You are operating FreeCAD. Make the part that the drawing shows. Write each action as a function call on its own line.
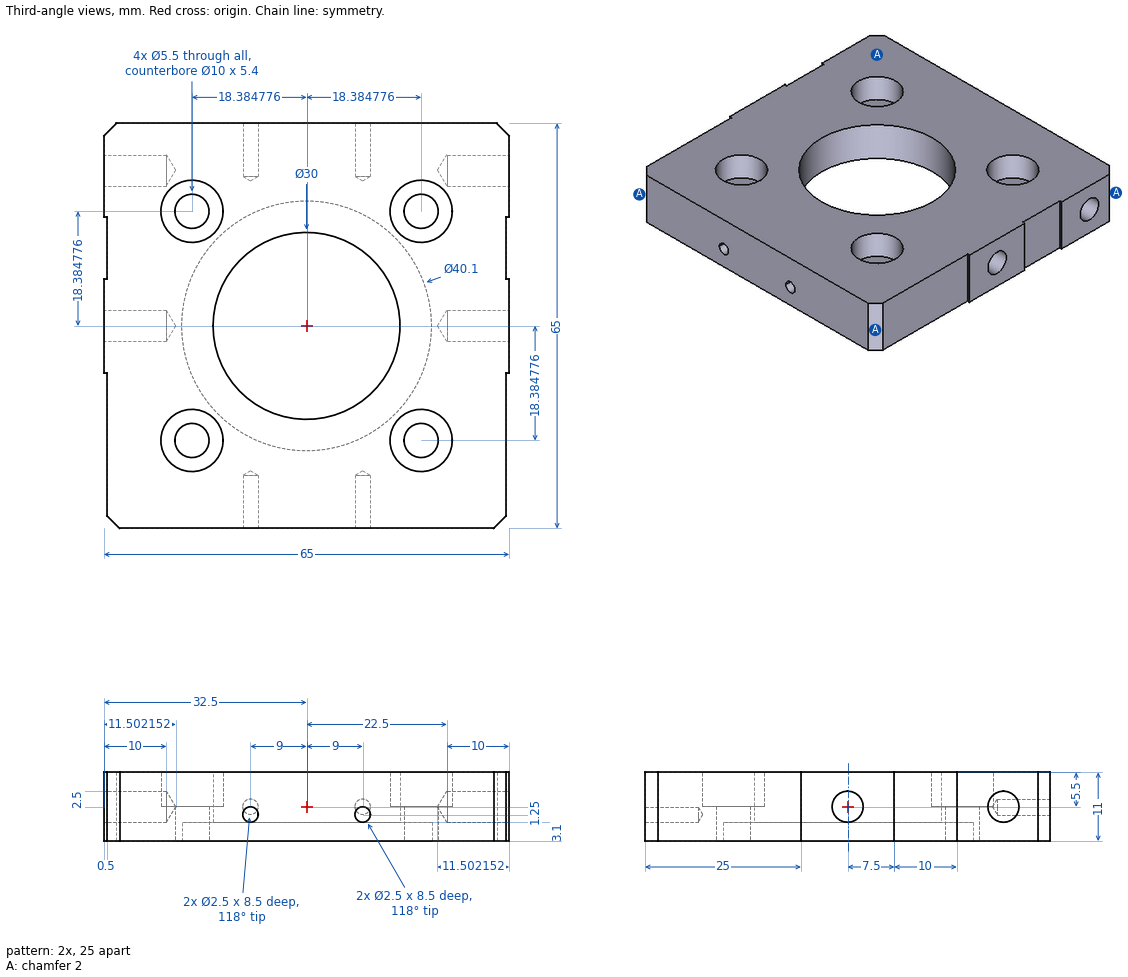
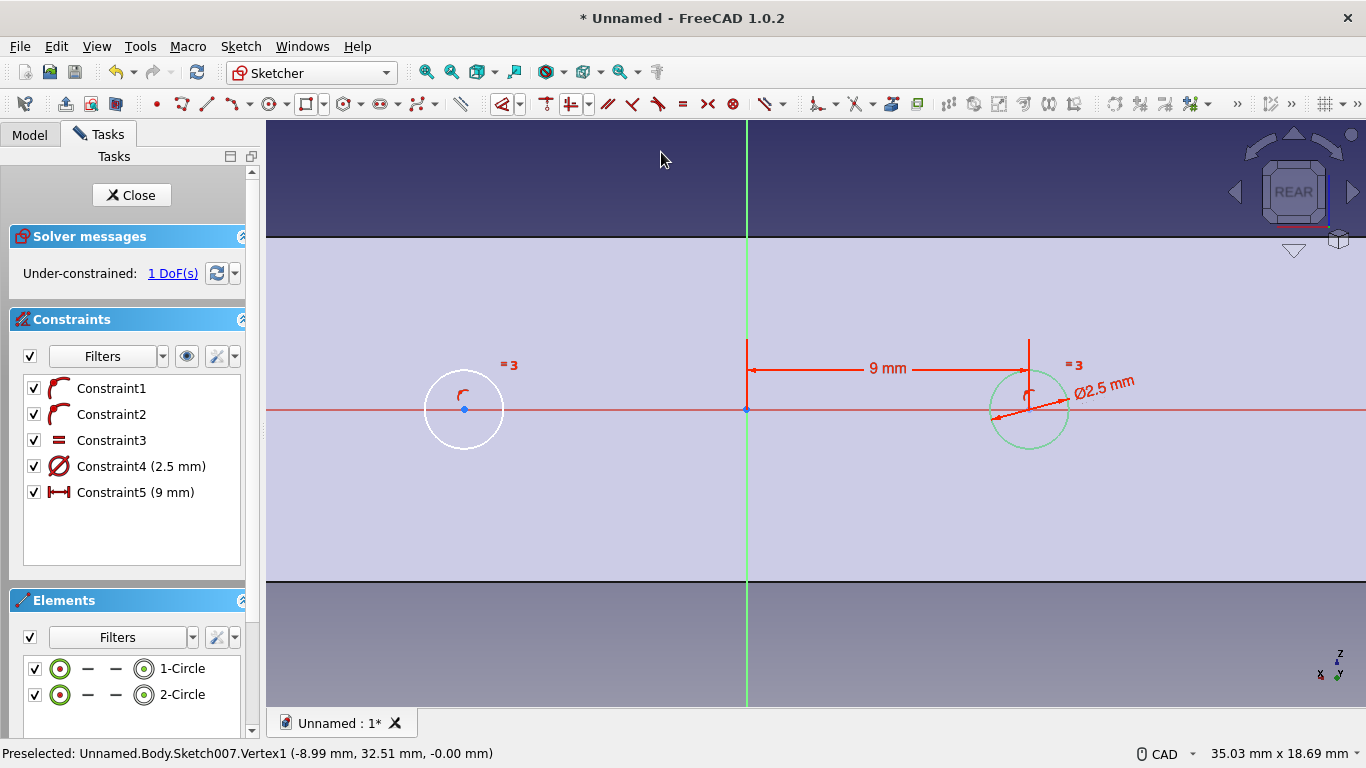
click(464, 410)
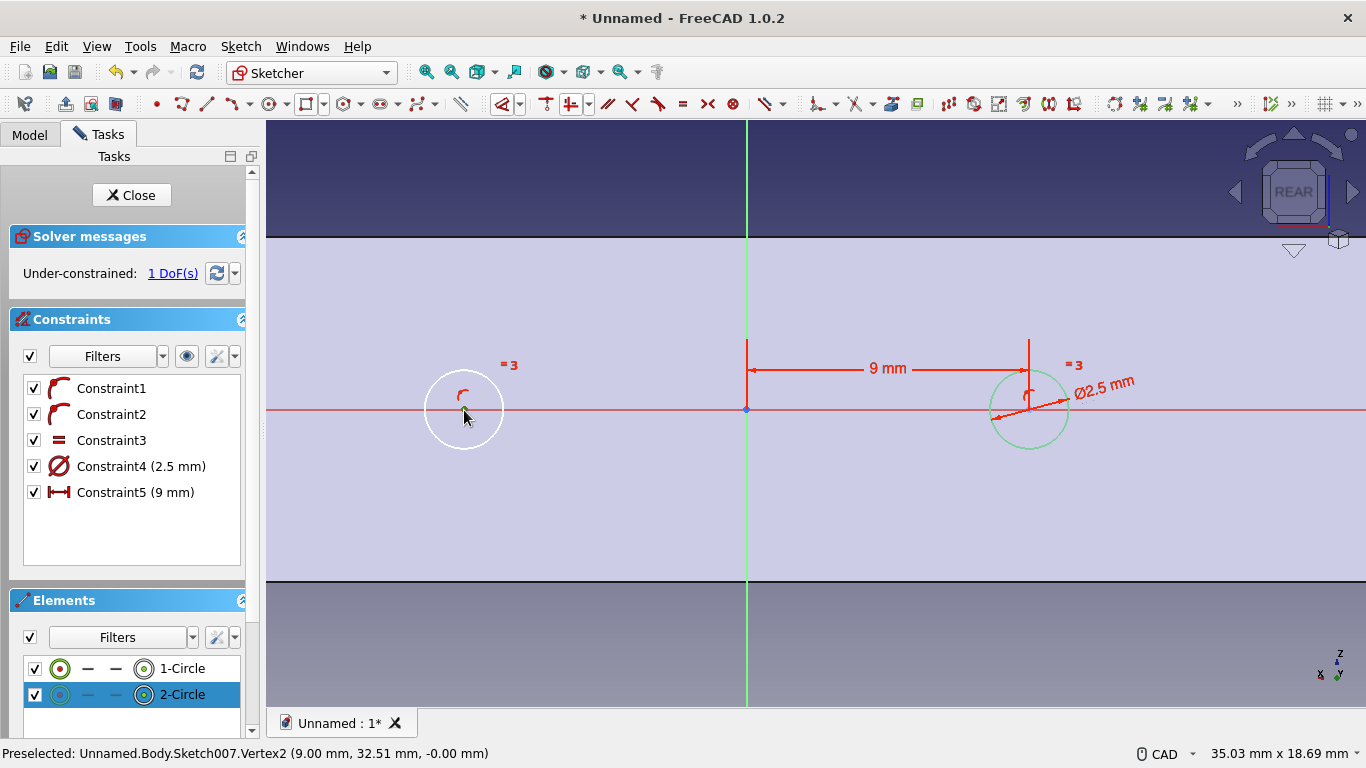
click(520, 104)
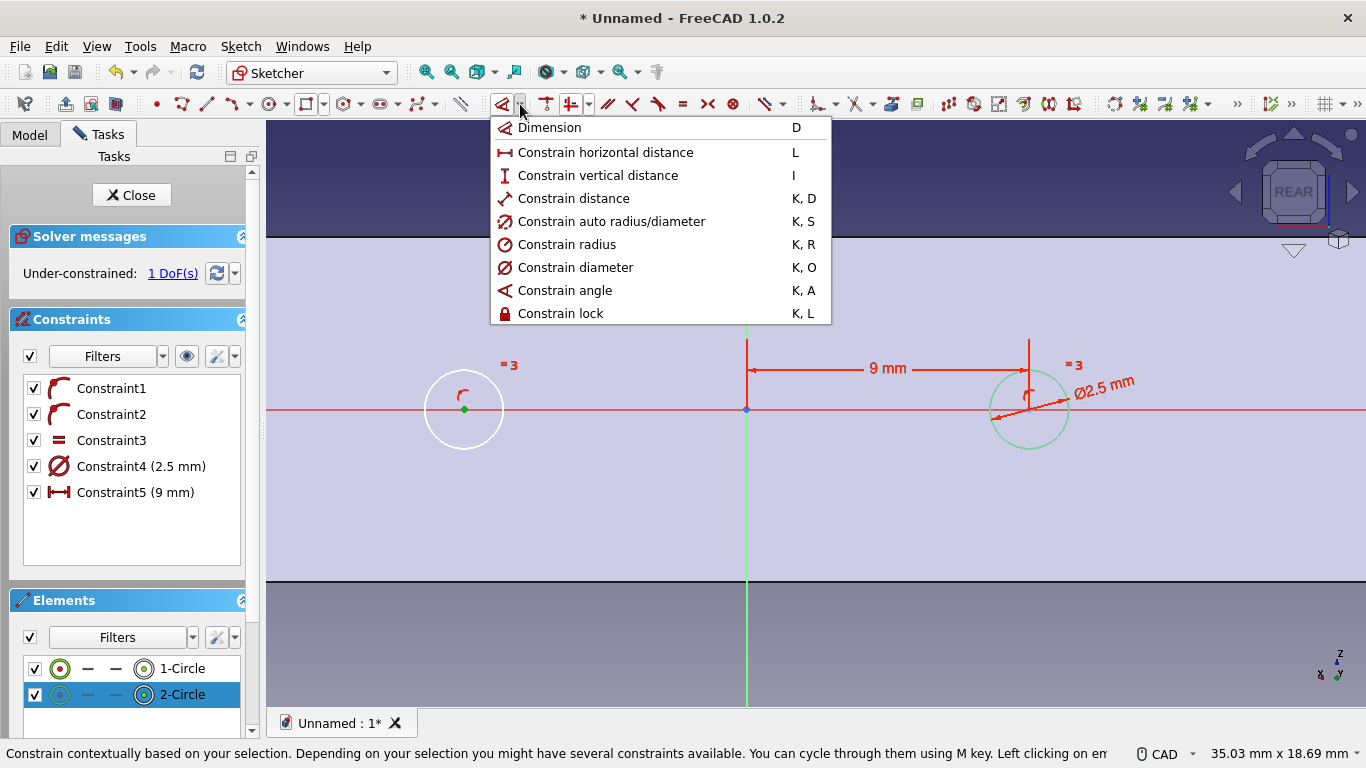
click(661, 152)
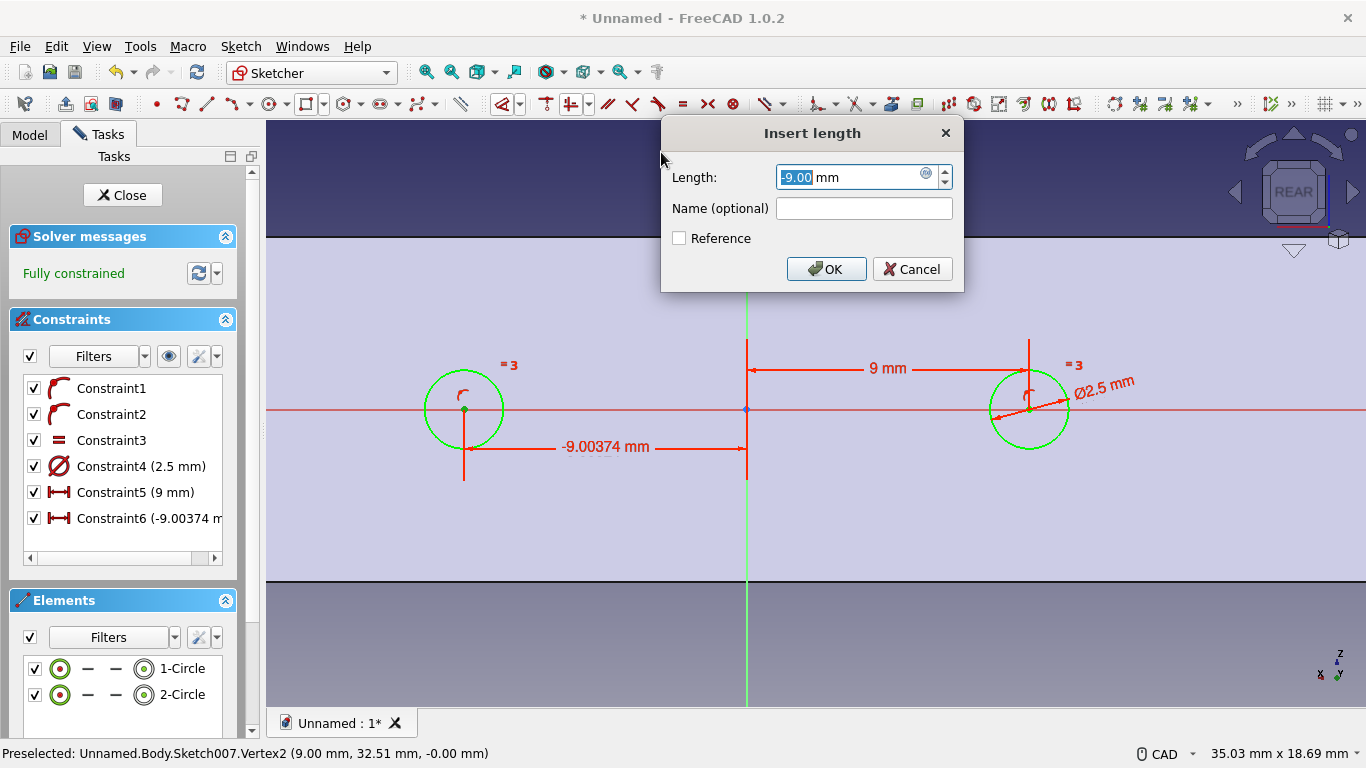
text(-9)
key(Return)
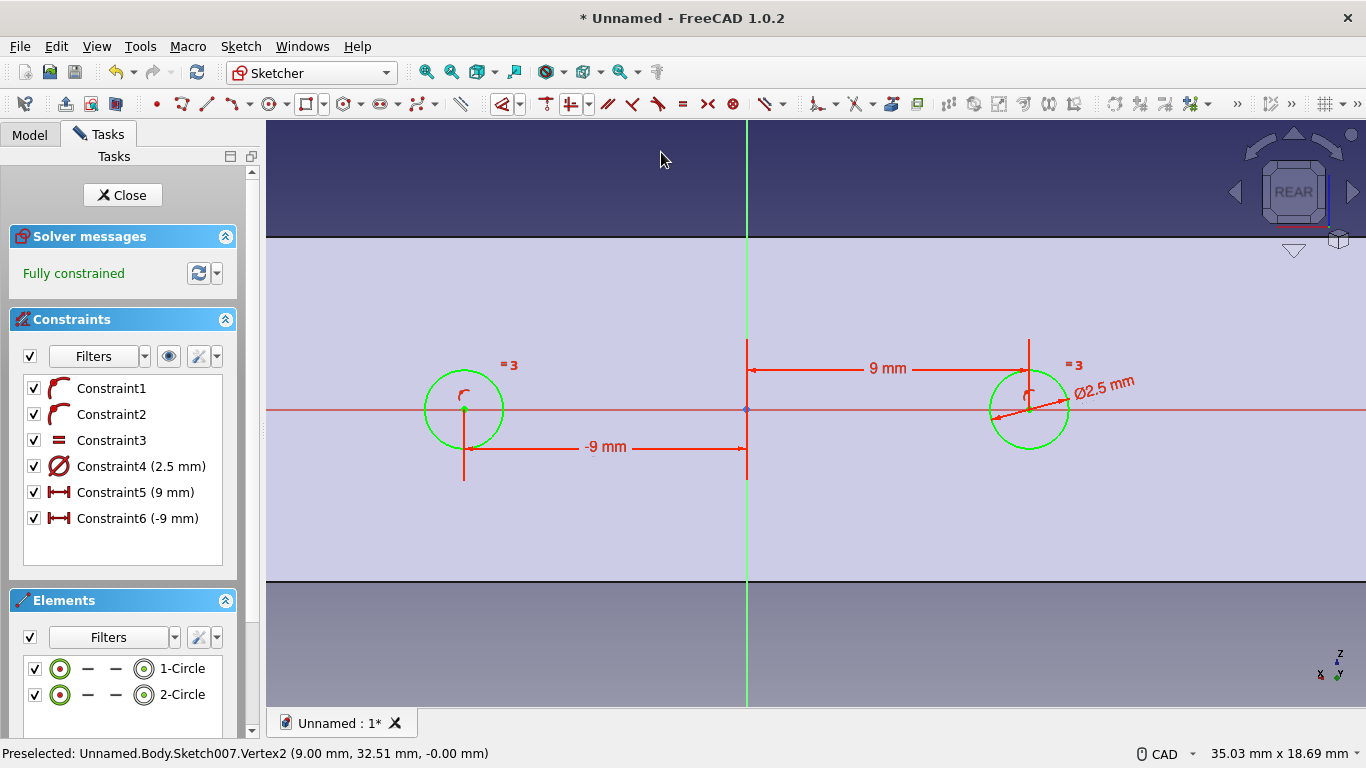
click(123, 195)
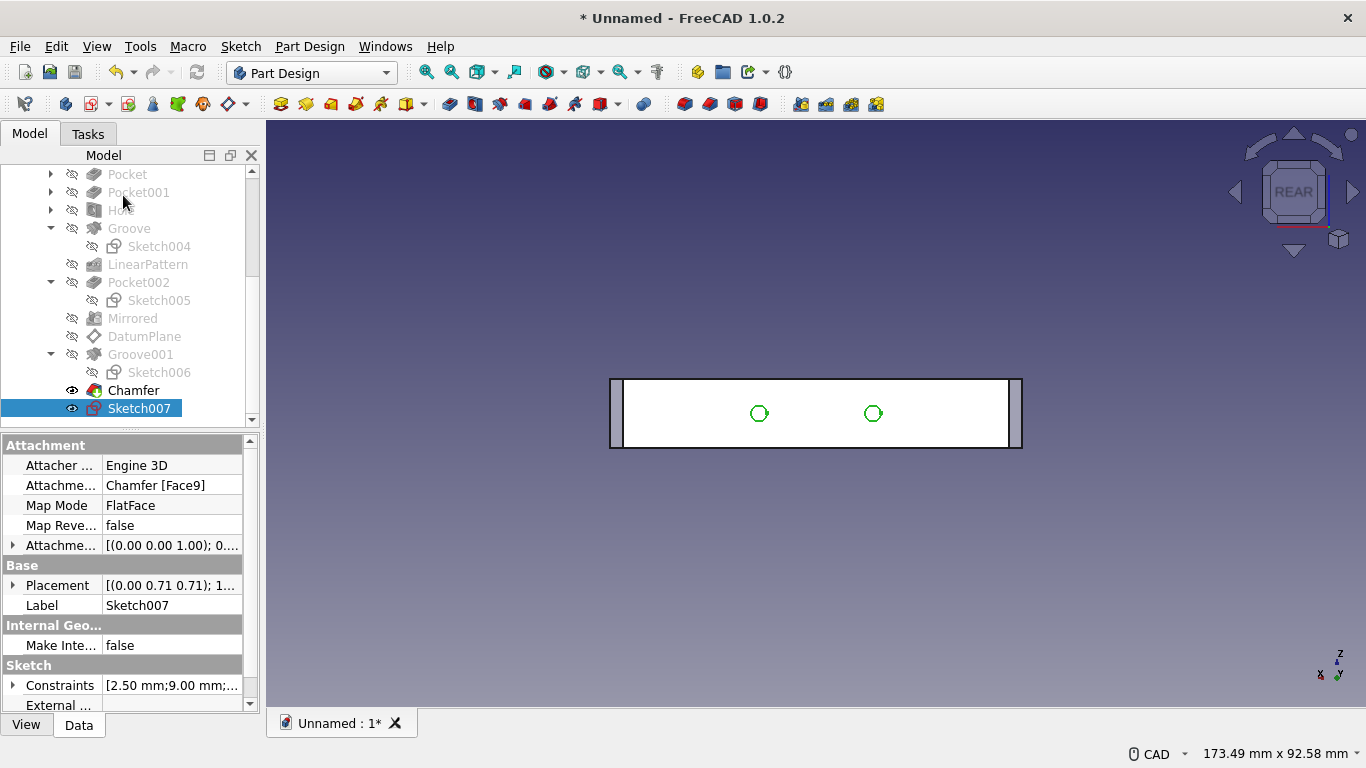
click(475, 104)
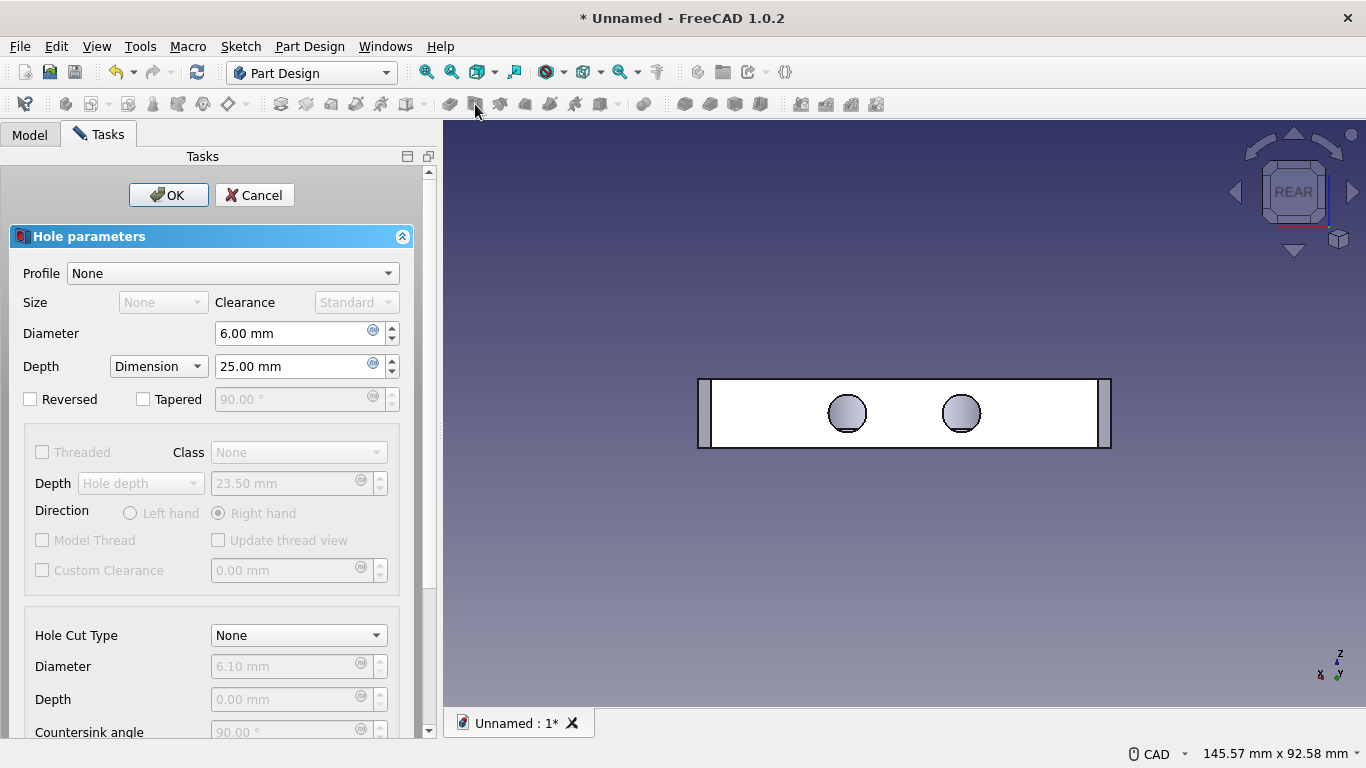
triple_click(300, 334)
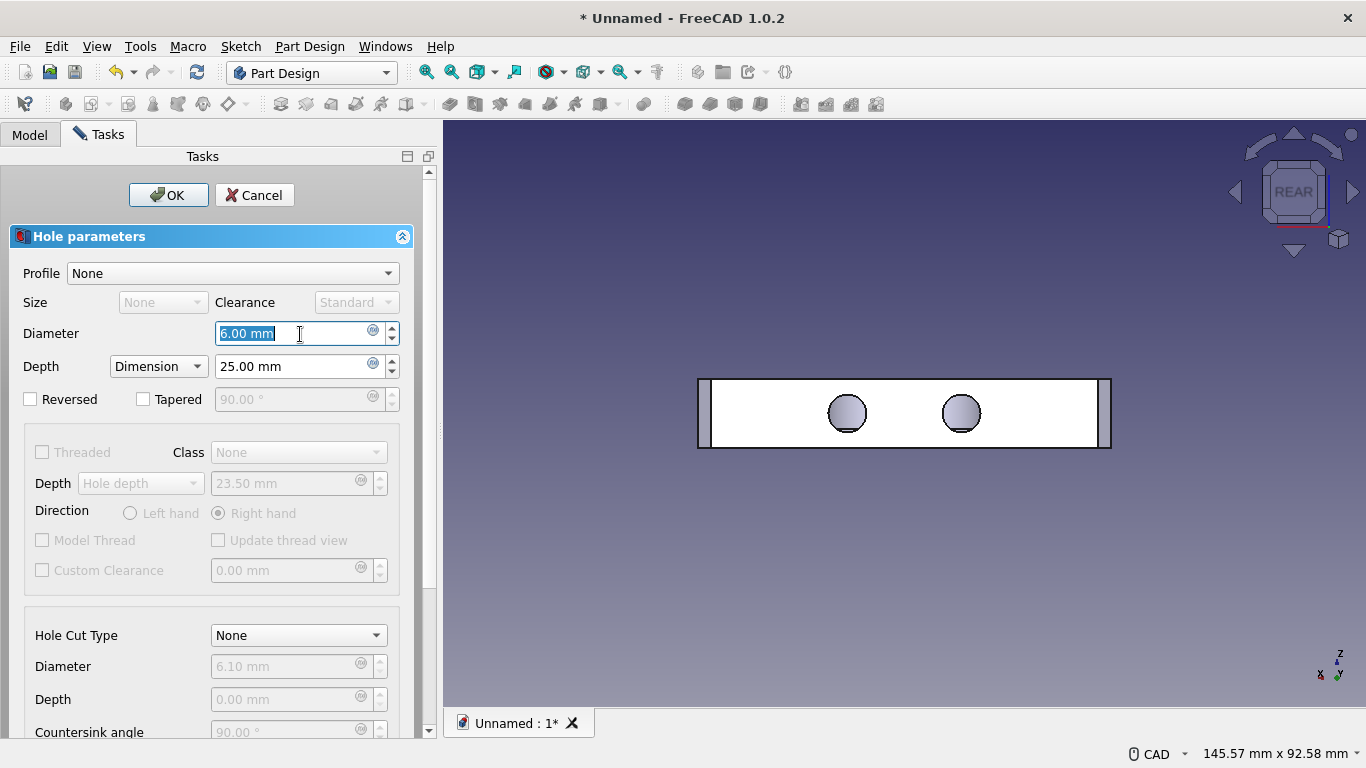
text(2.5)
key(Tab)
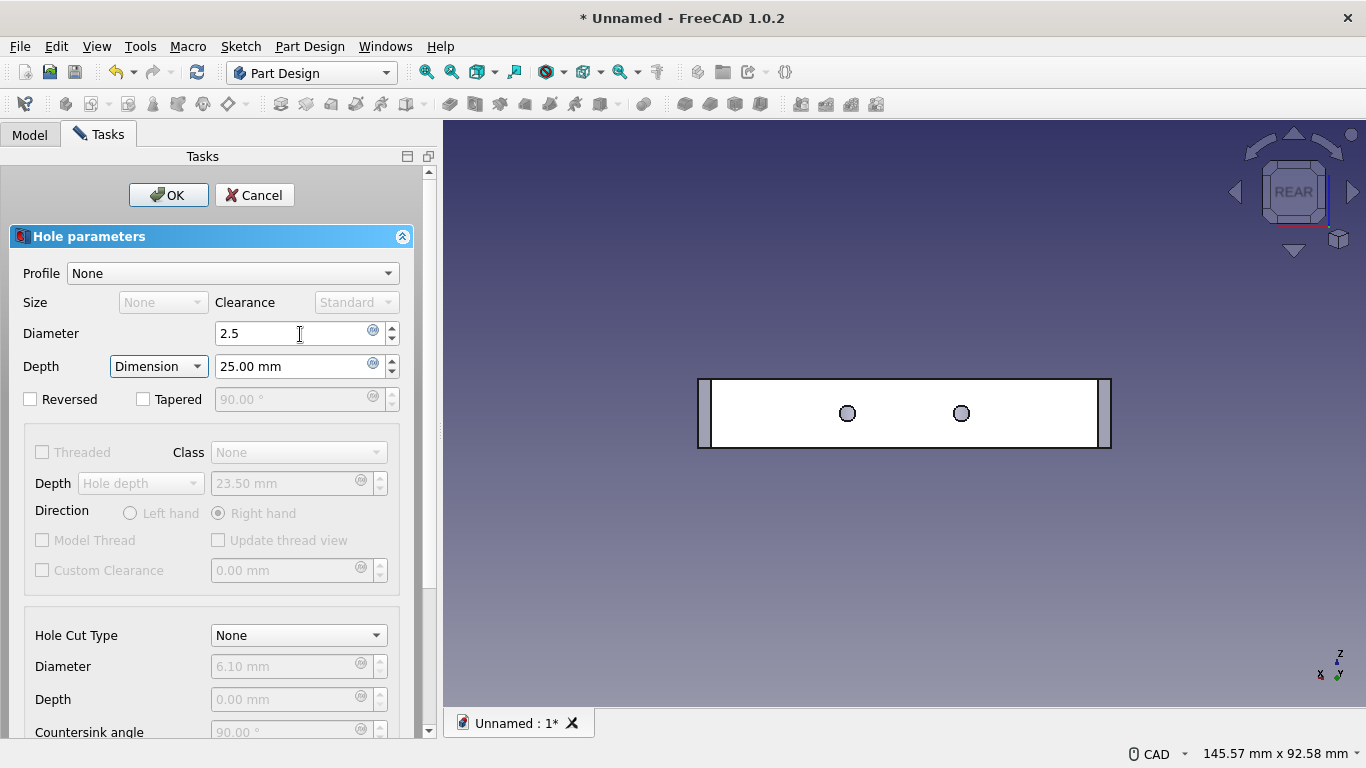
triple_click(300, 366)